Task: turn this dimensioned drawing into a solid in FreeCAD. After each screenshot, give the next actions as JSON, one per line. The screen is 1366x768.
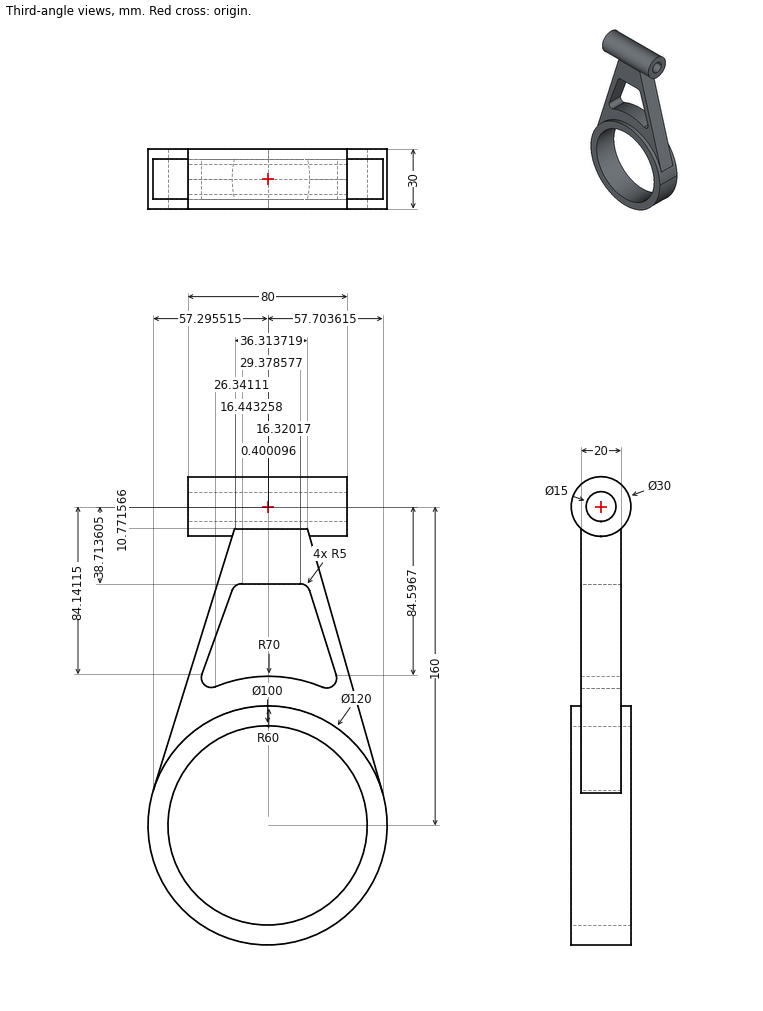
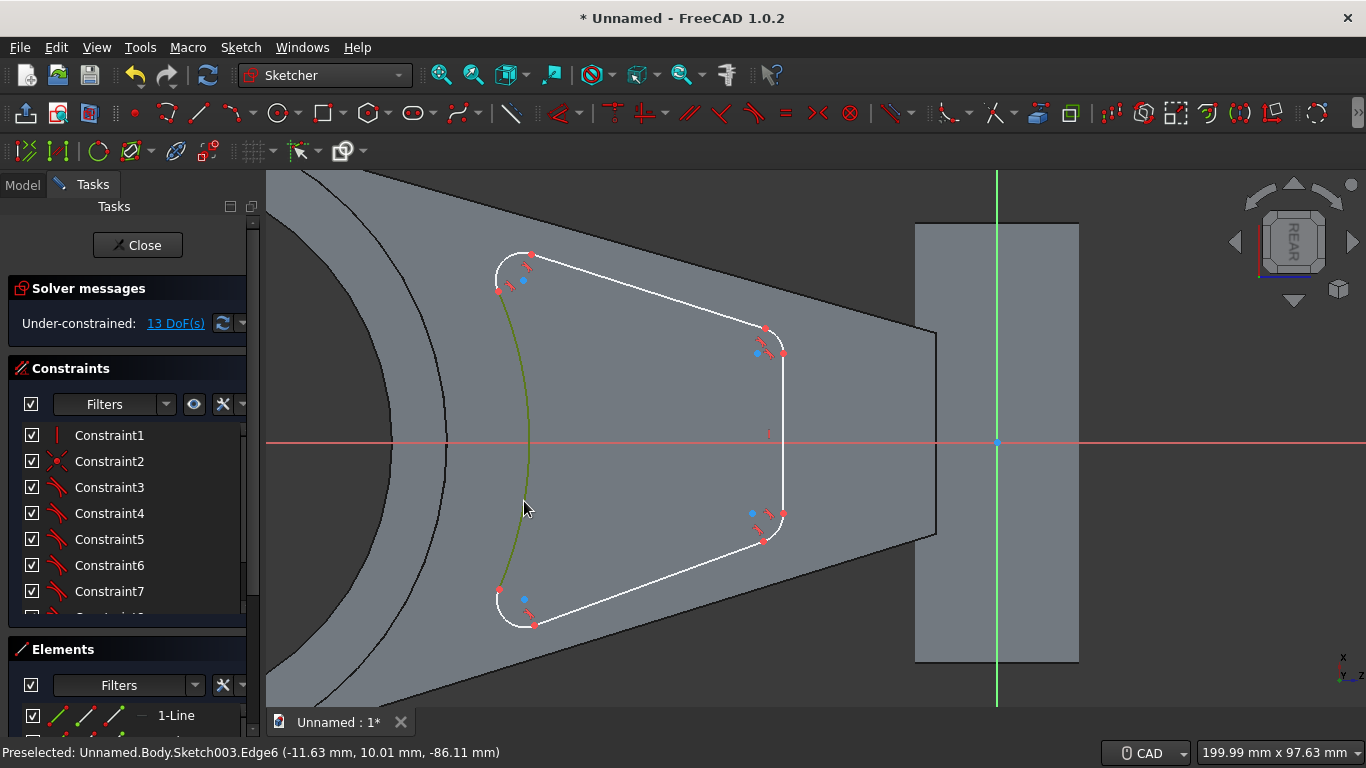
{"action": "left_click", "coordinate": [498, 608]}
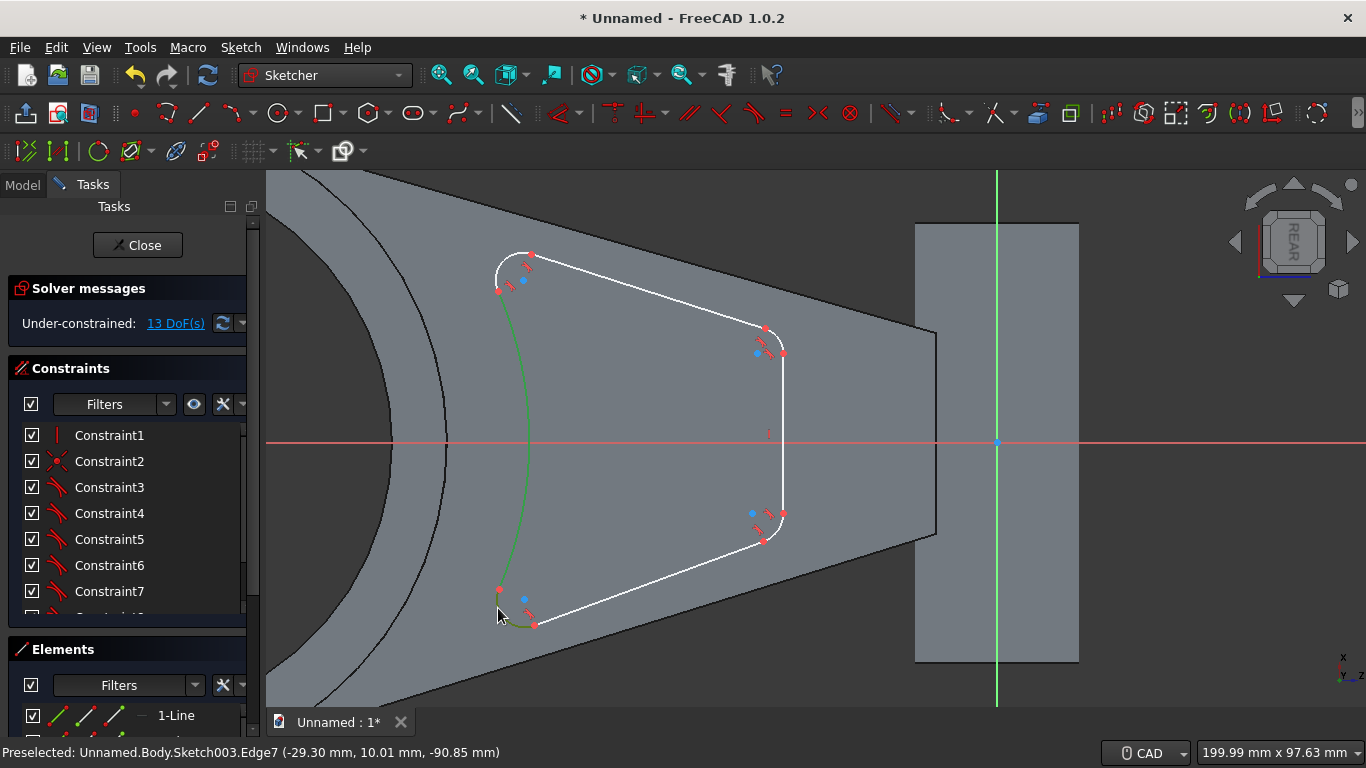
{"action": "left_click", "coordinate": [754, 114]}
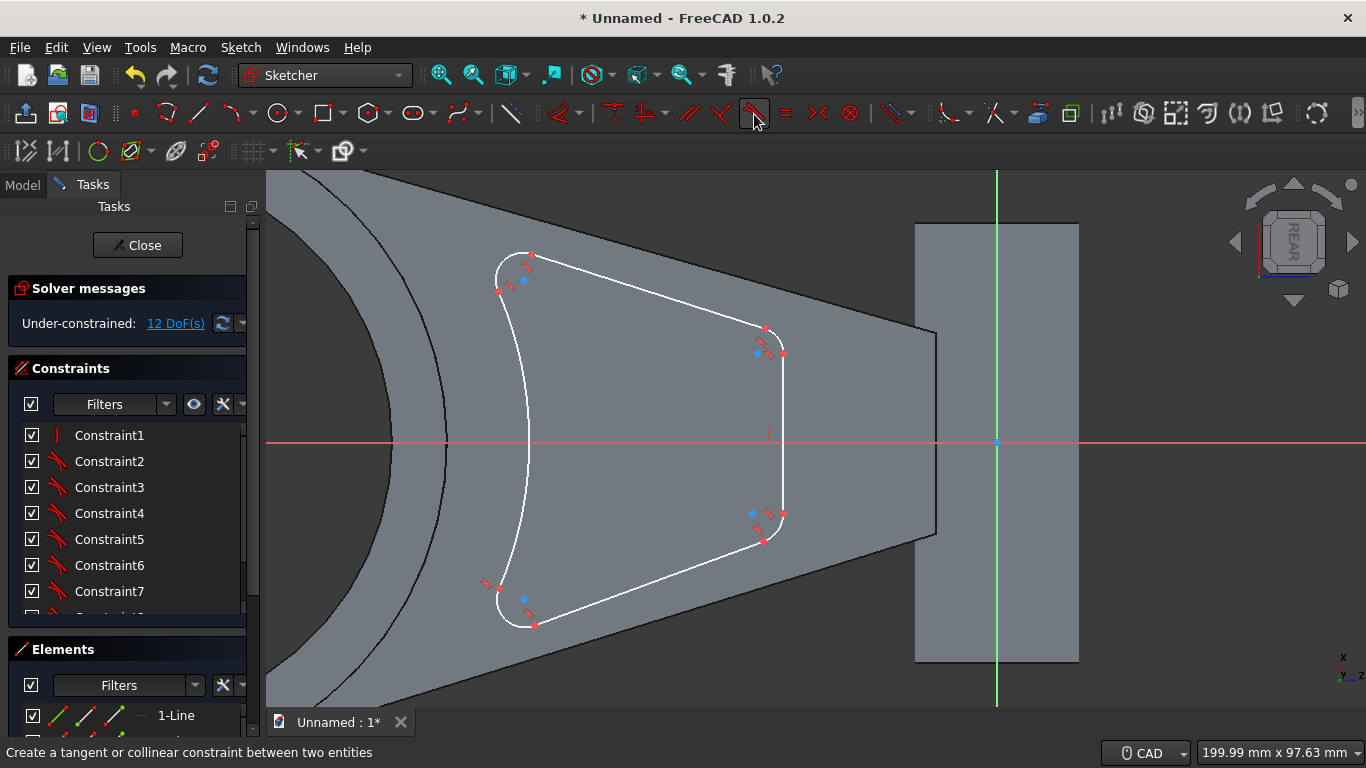
{"action": "scroll", "coordinate": [781, 344], "scroll_direction": "up", "scroll_amount": 2}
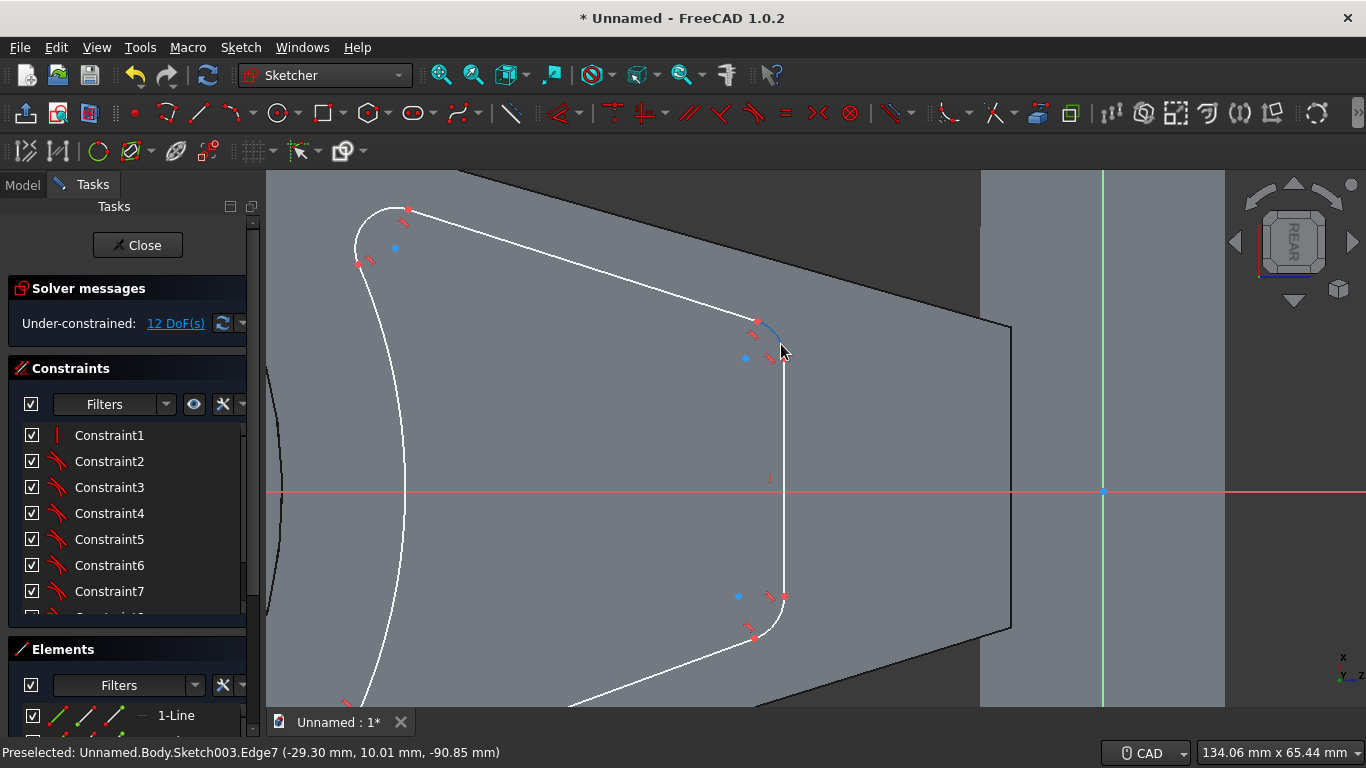
{"action": "left_click", "coordinate": [782, 344]}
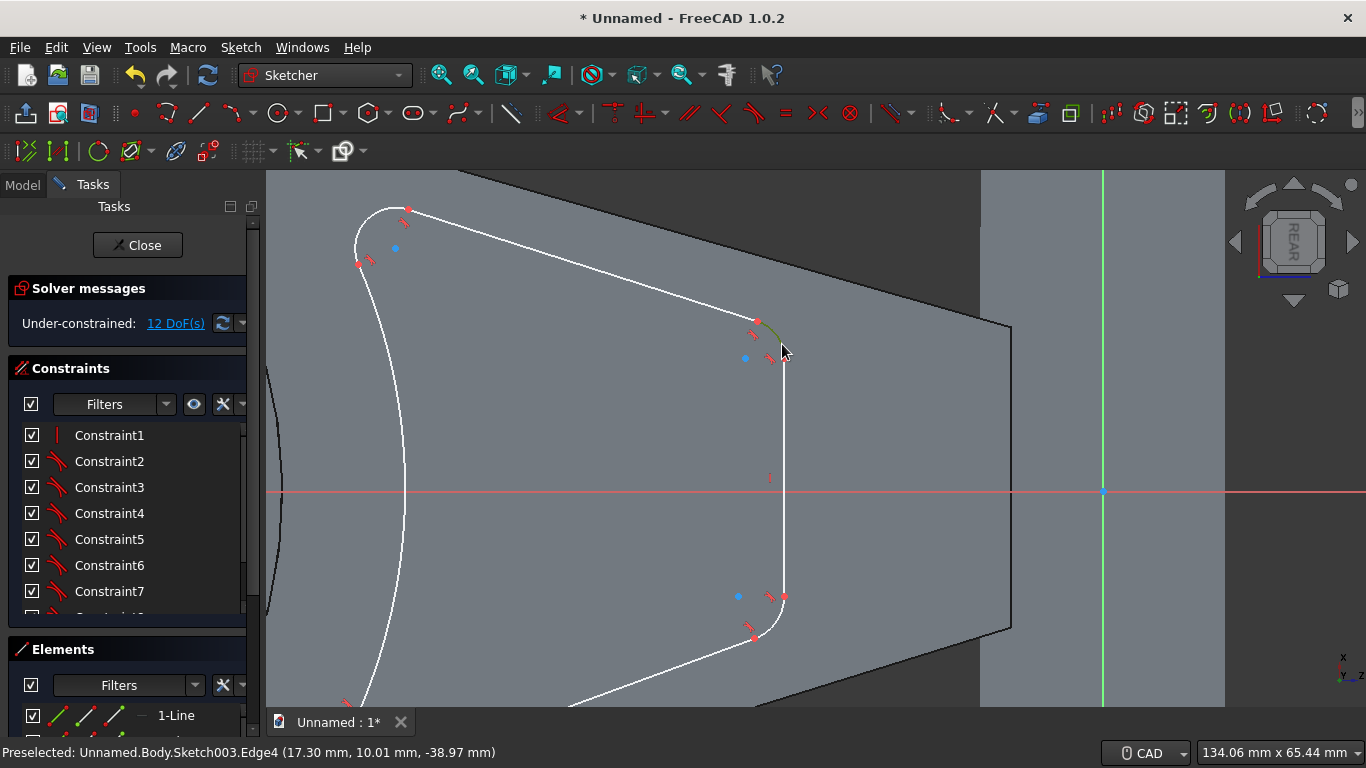
{"action": "left_click", "coordinate": [381, 211]}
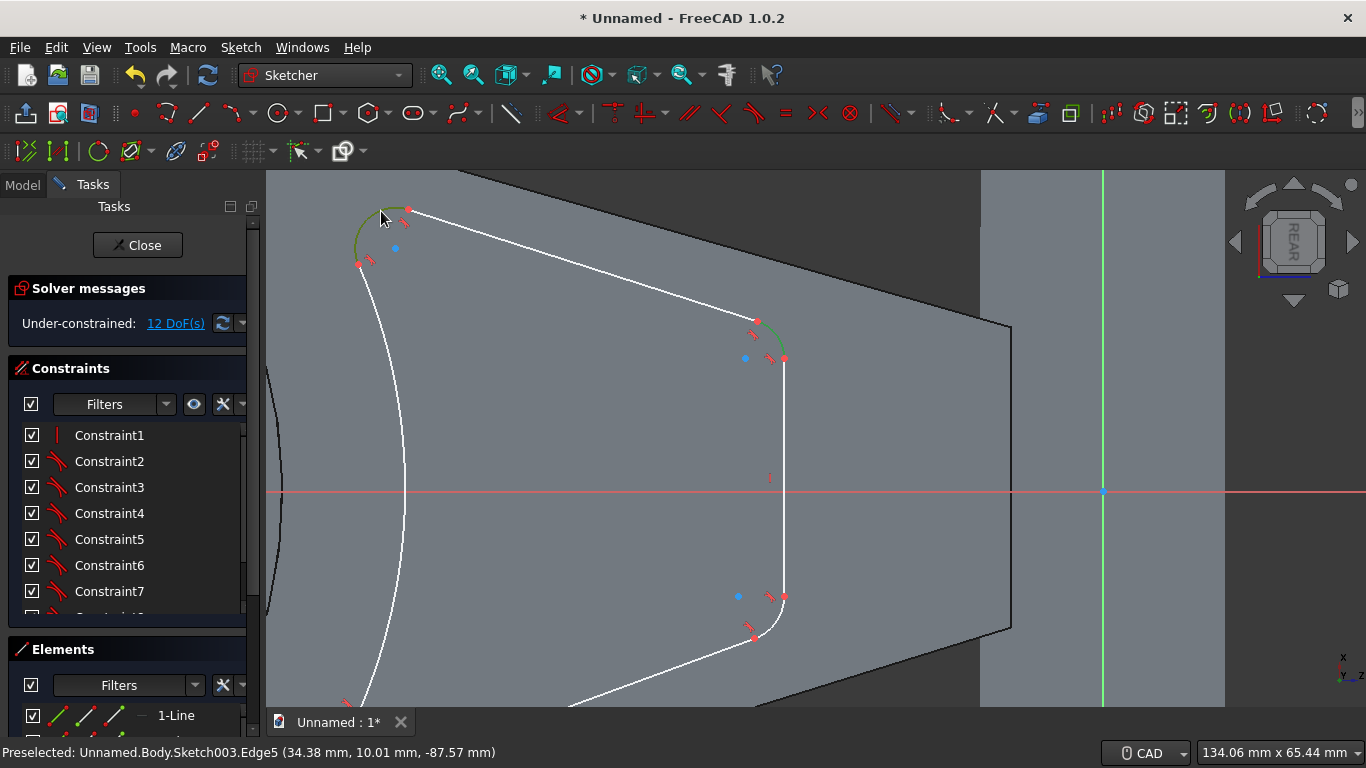
{"action": "scroll", "coordinate": [781, 343], "scroll_direction": "down", "scroll_amount": 2}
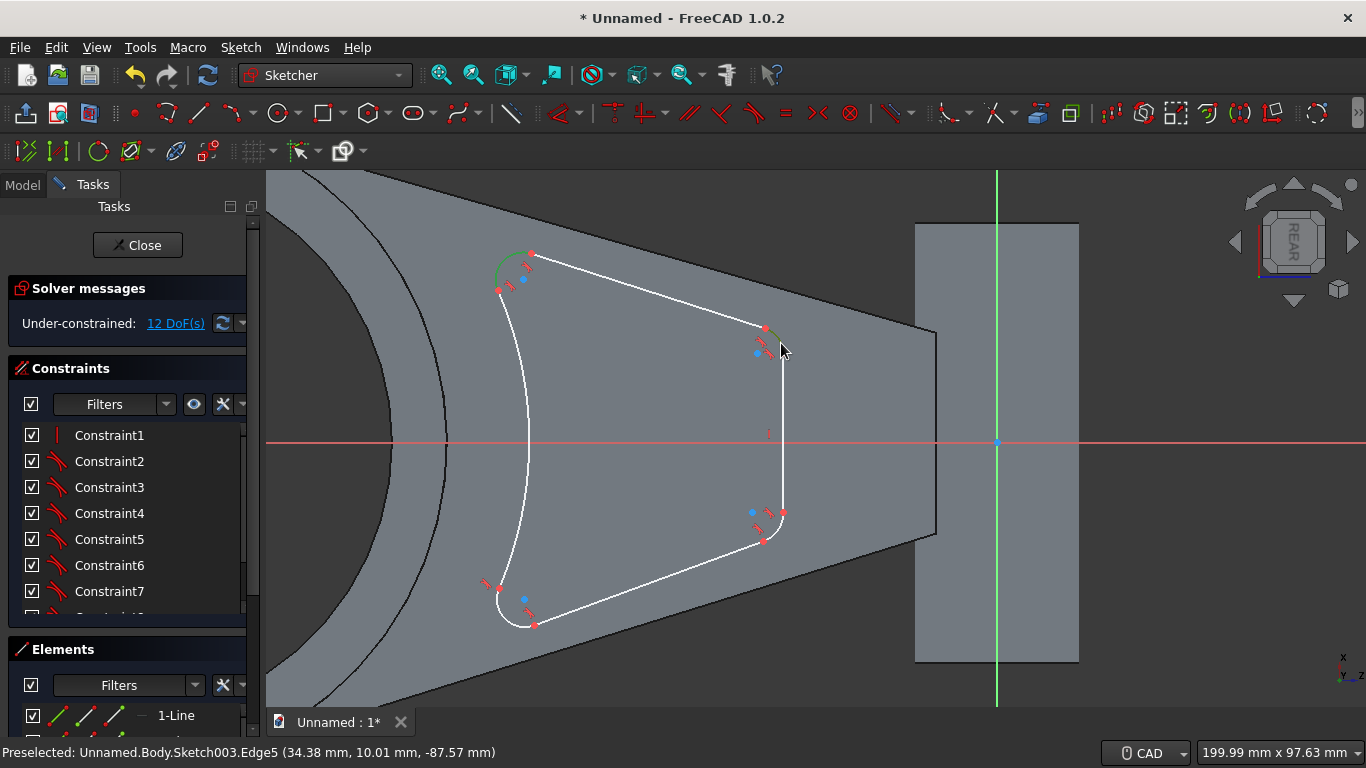
{"action": "left_click", "coordinate": [498, 607]}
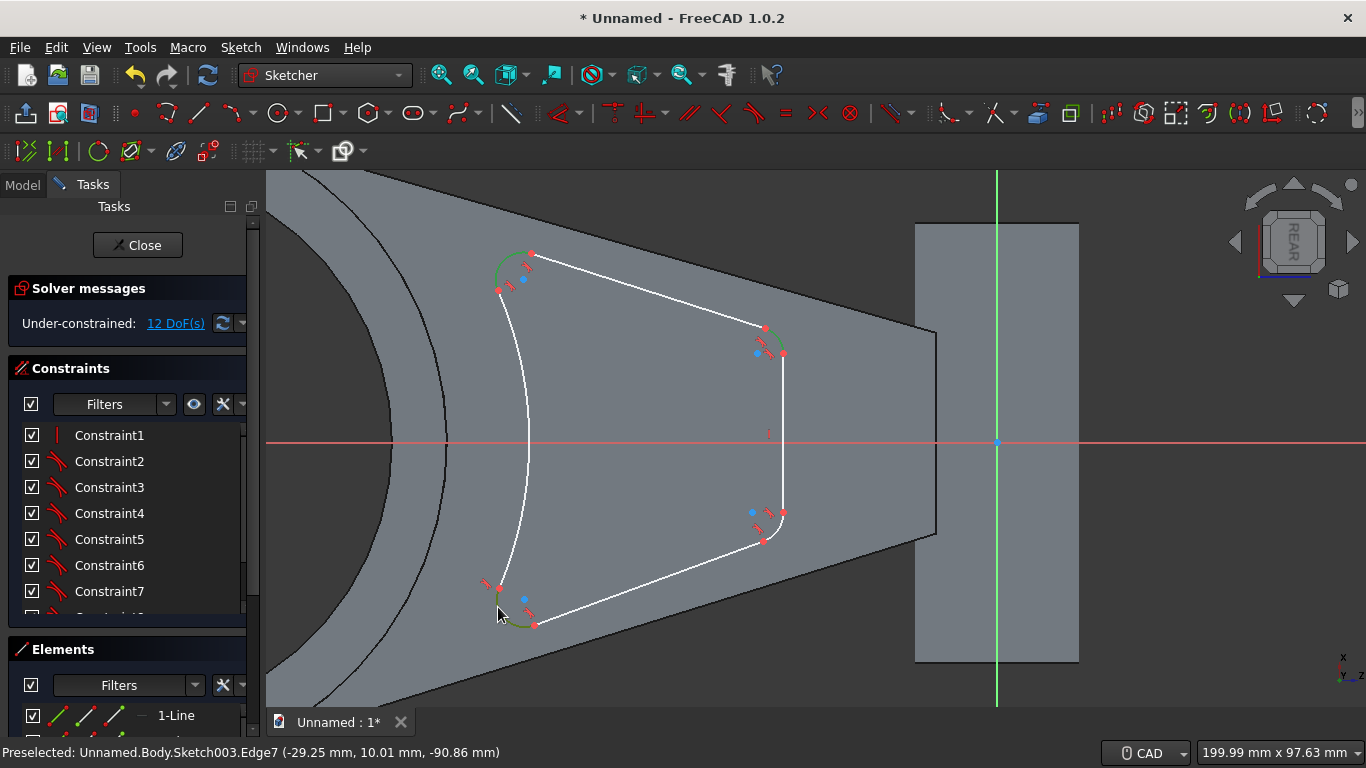
{"action": "scroll", "coordinate": [773, 536], "scroll_direction": "up", "scroll_amount": 2}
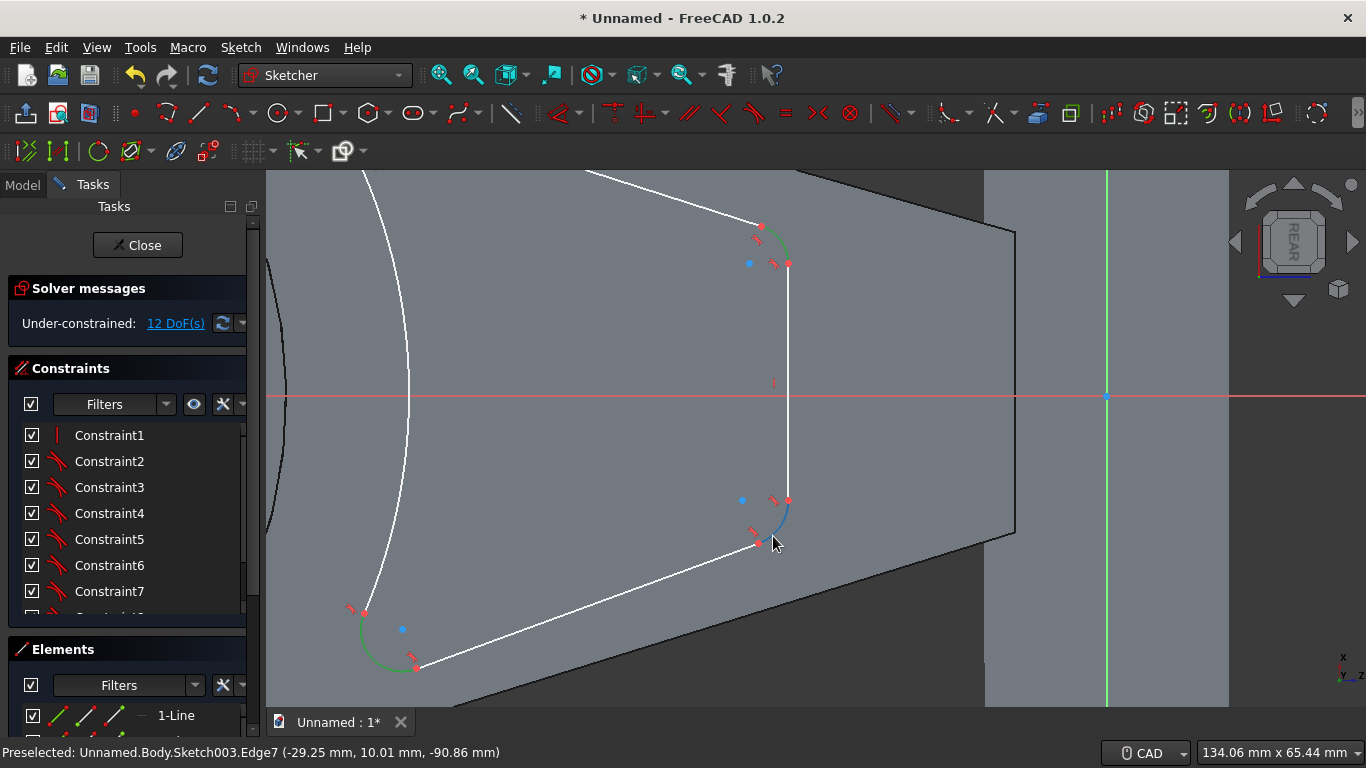
{"action": "left_click", "coordinate": [773, 535]}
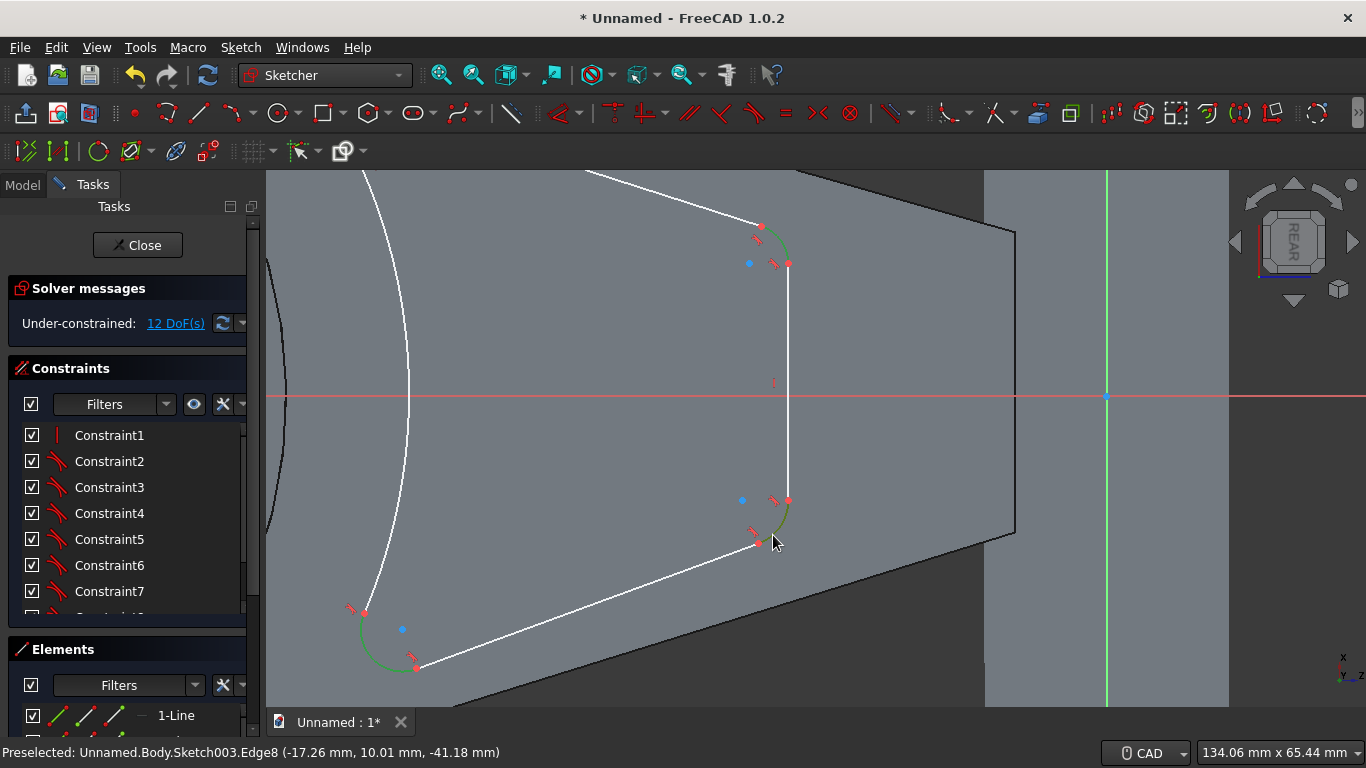
{"action": "left_click", "coordinate": [786, 114]}